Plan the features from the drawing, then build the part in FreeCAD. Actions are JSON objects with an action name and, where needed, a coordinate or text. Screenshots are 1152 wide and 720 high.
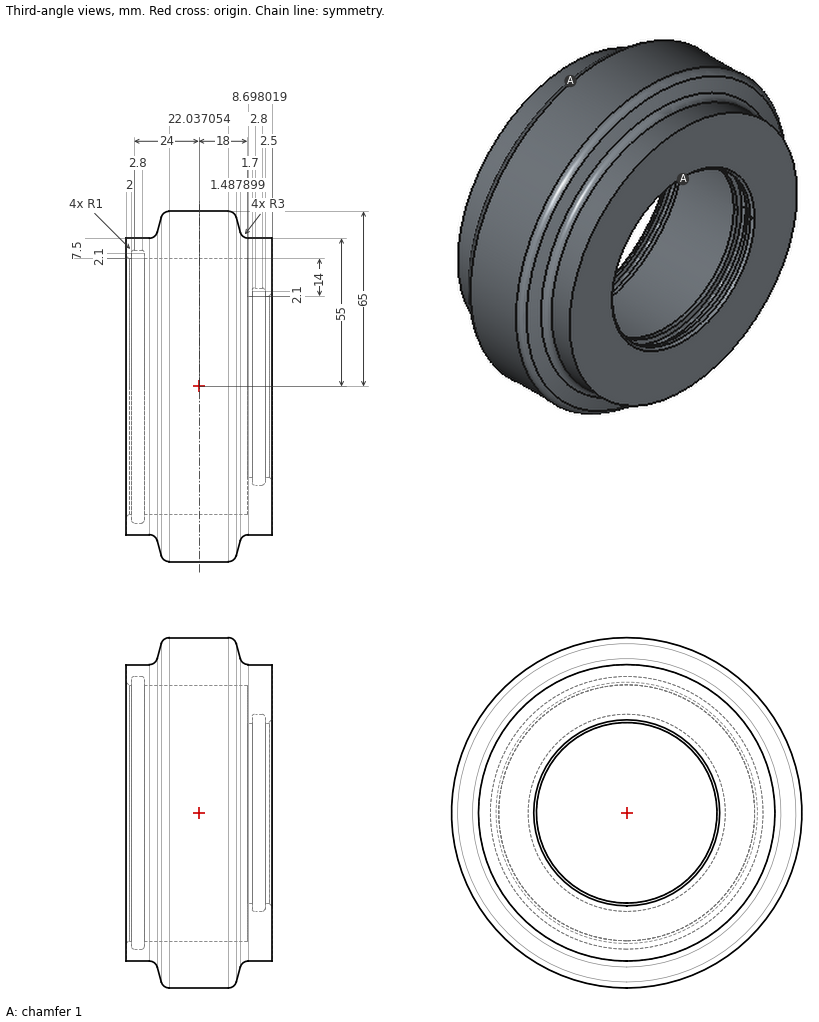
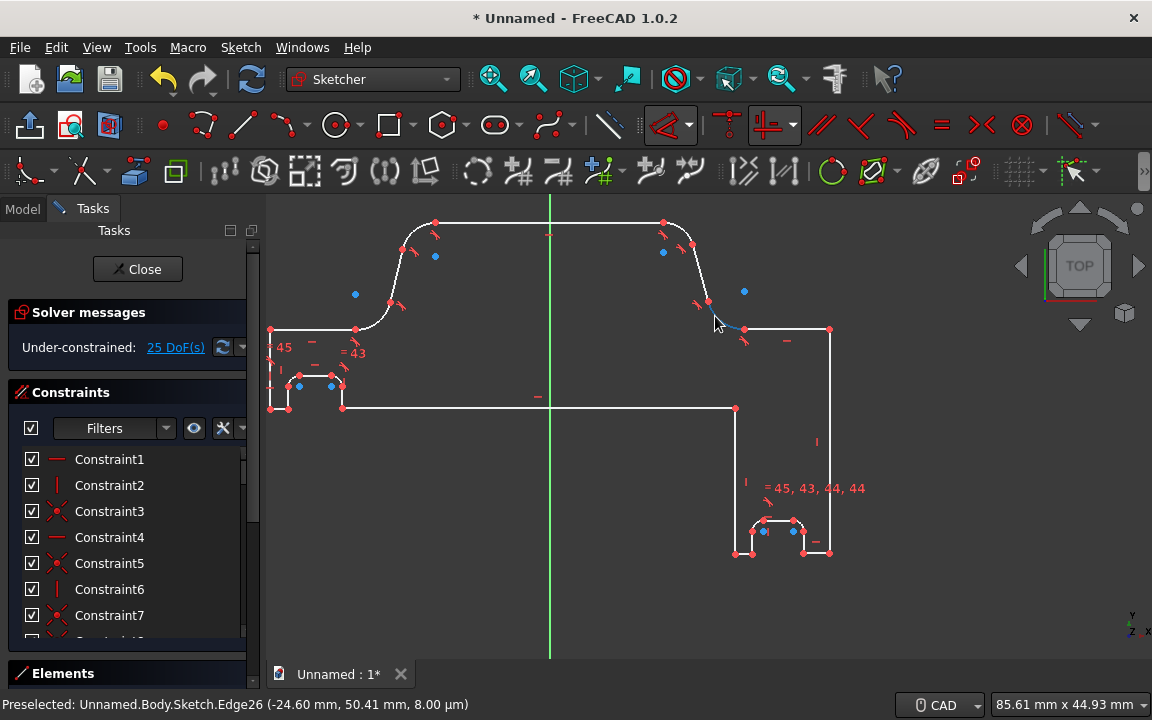
{"action": "left_click", "coordinate": [715, 315]}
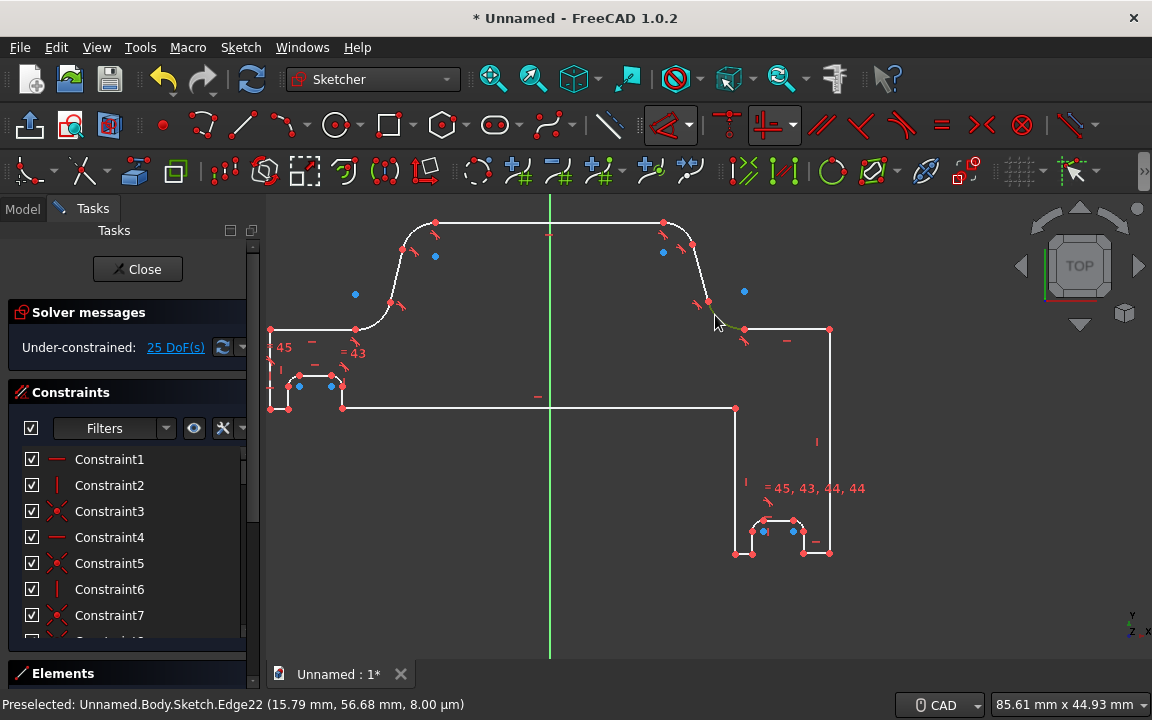
{"action": "left_click", "coordinate": [688, 235]}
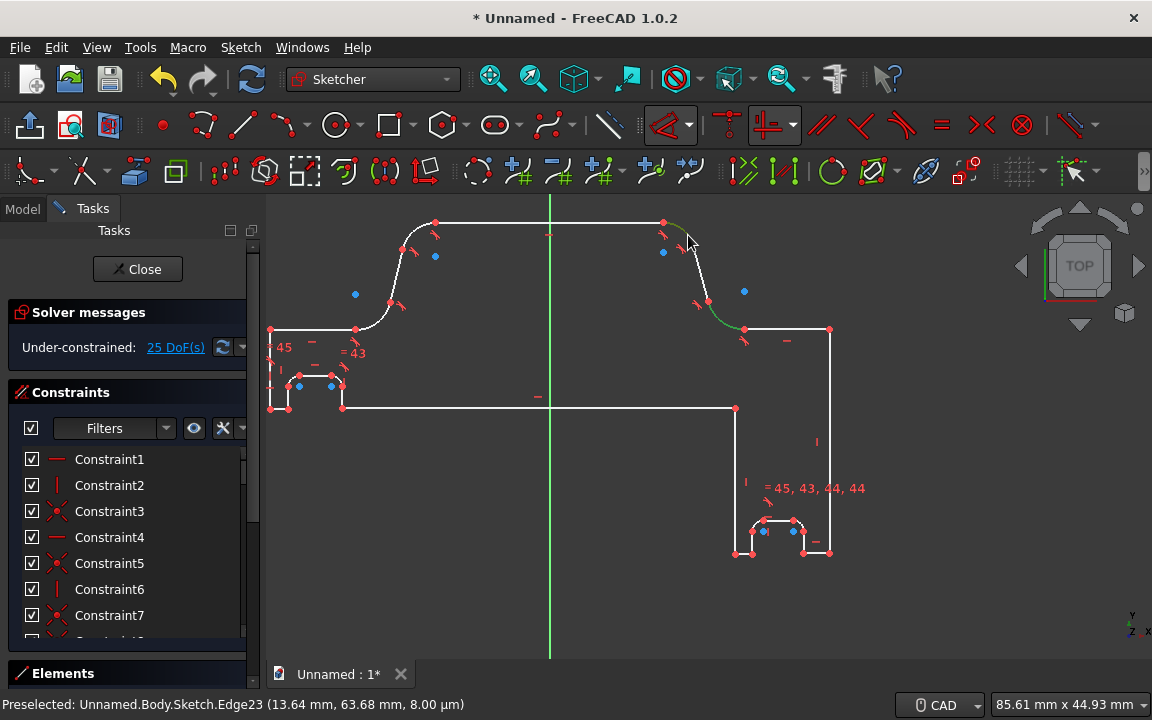
{"action": "left_click", "coordinate": [423, 226]}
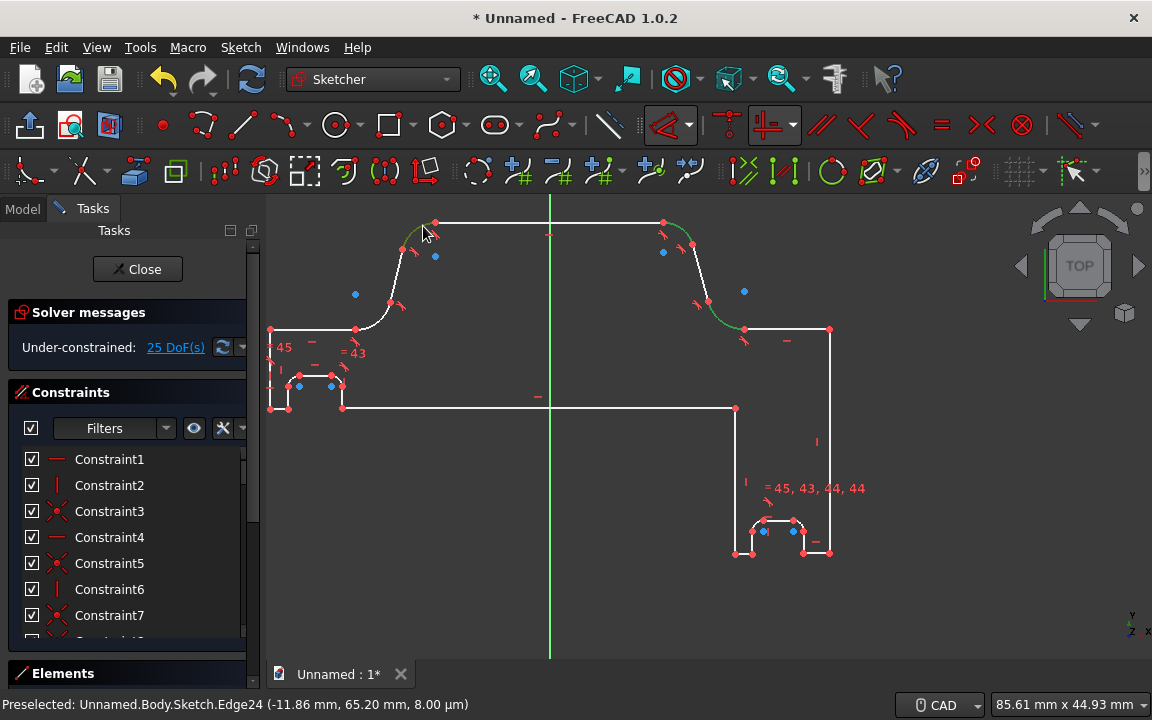
{"action": "left_click", "coordinate": [370, 327]}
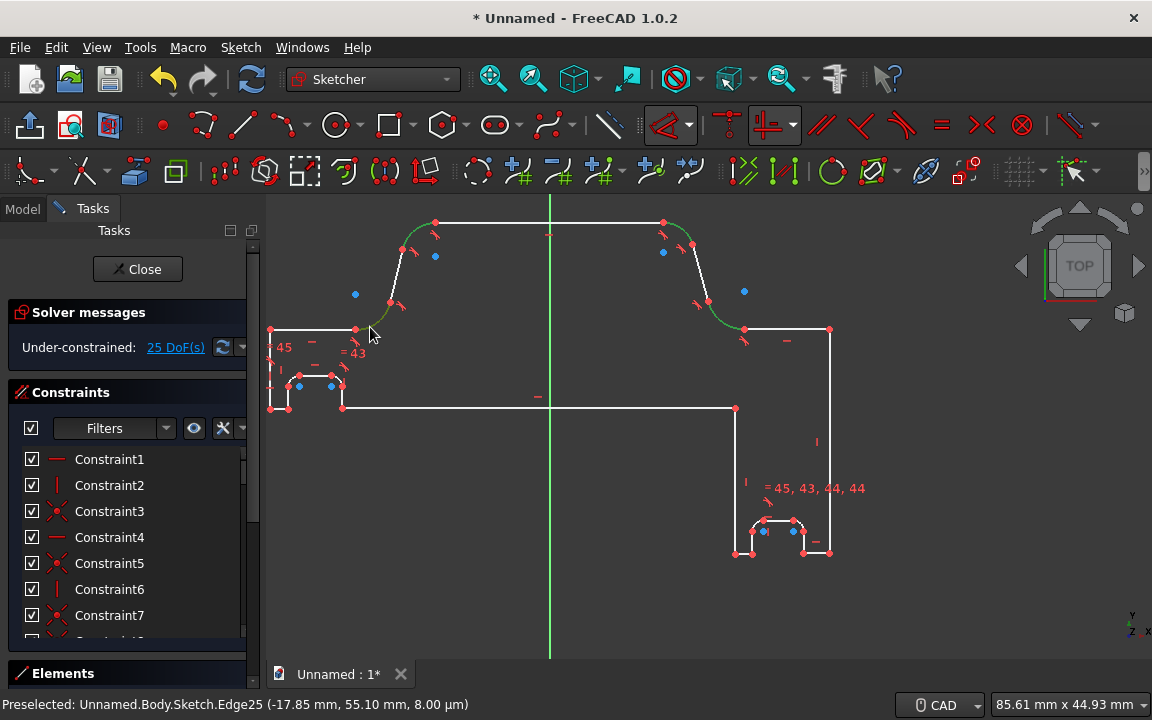
{"action": "left_click", "coordinate": [942, 126]}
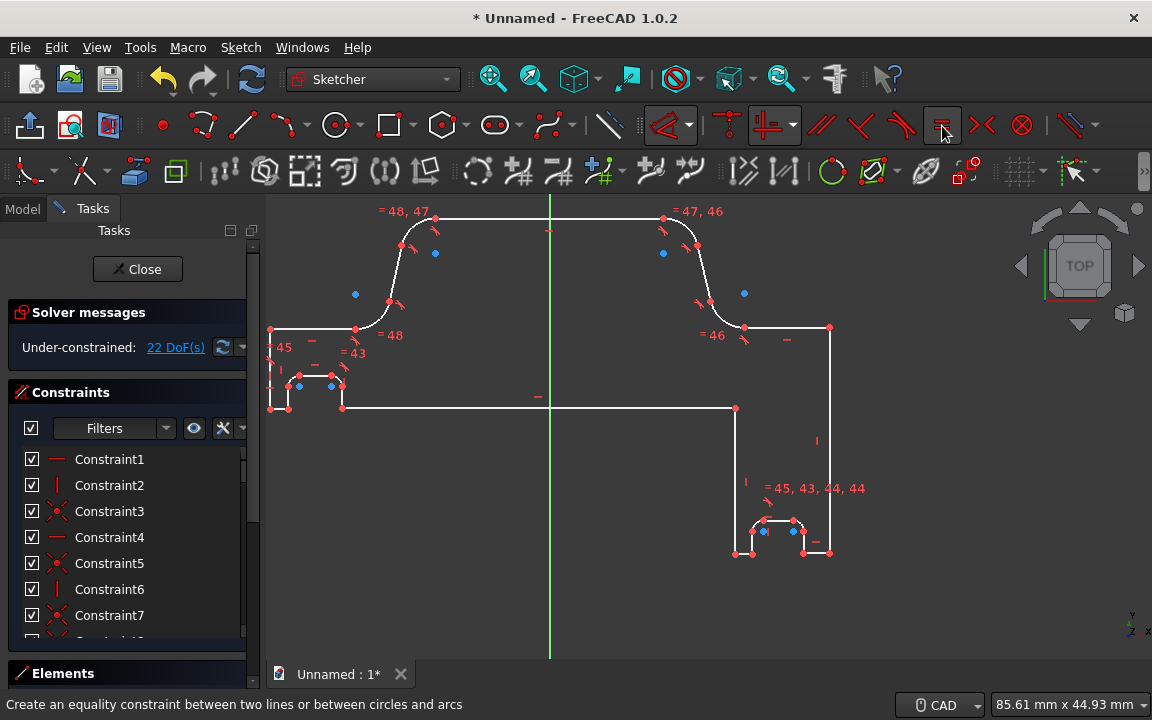
{"action": "left_click", "coordinate": [745, 293]}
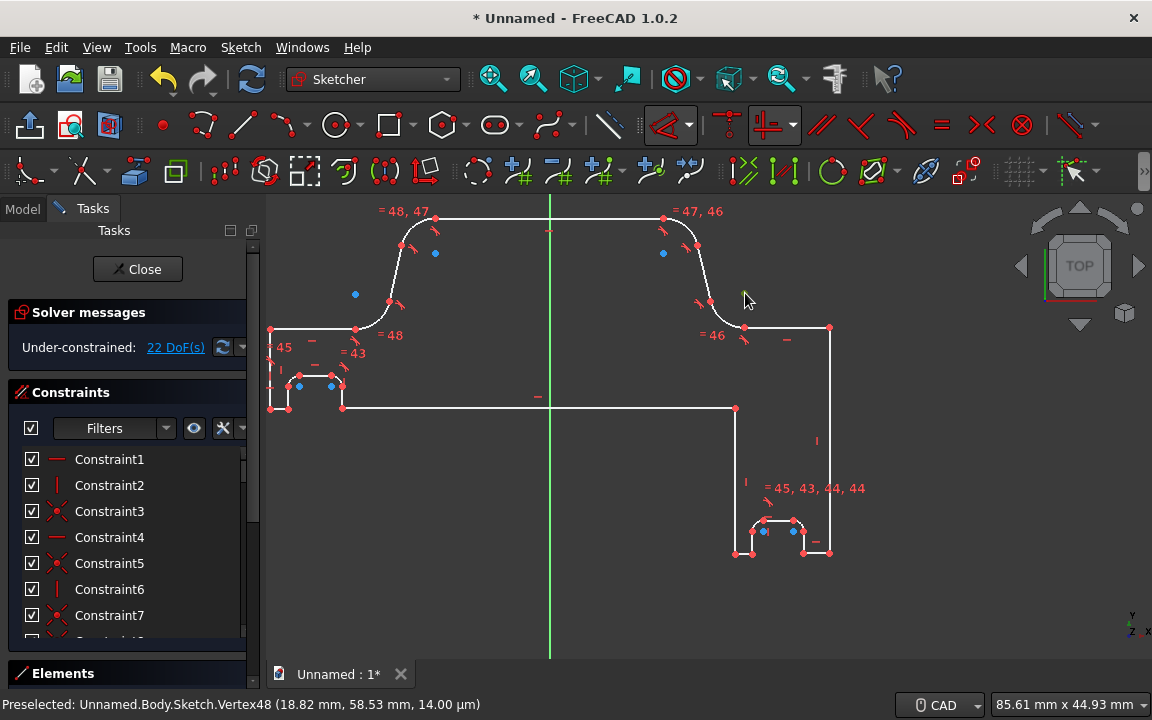
{"action": "left_click", "coordinate": [356, 294]}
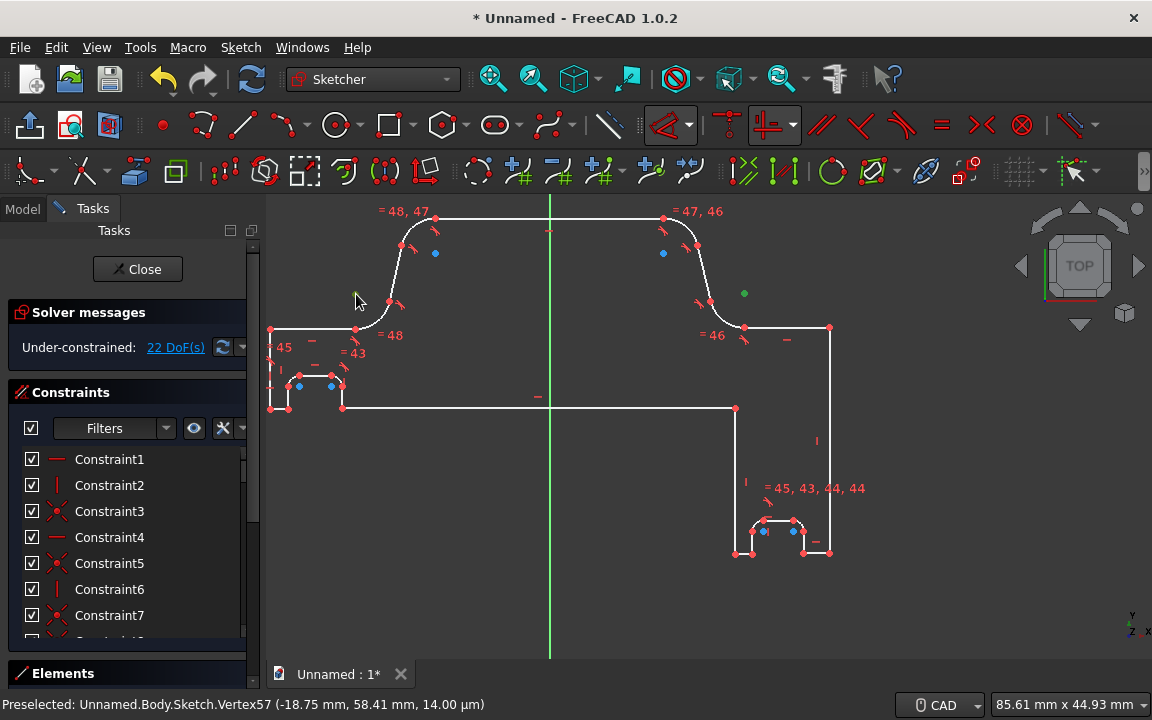
{"action": "left_click", "coordinate": [550, 602]}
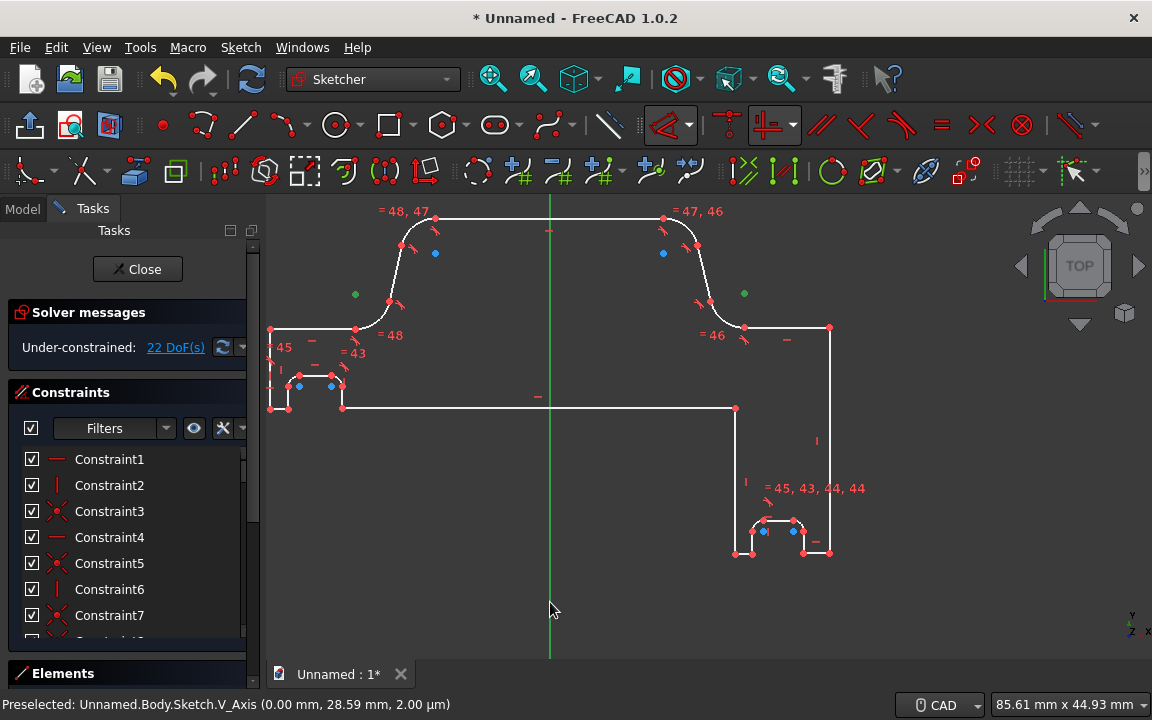
{"action": "key", "text": "s"}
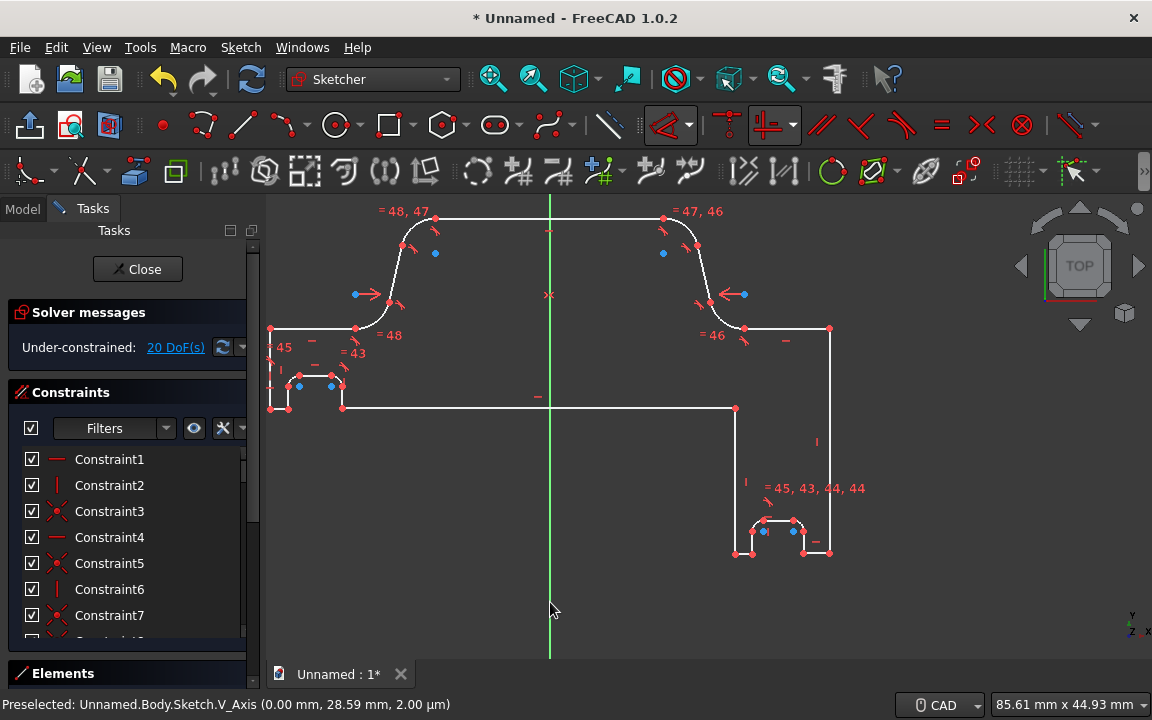
{"action": "scroll", "coordinate": [339, 379], "scroll_direction": "up", "scroll_amount": 7}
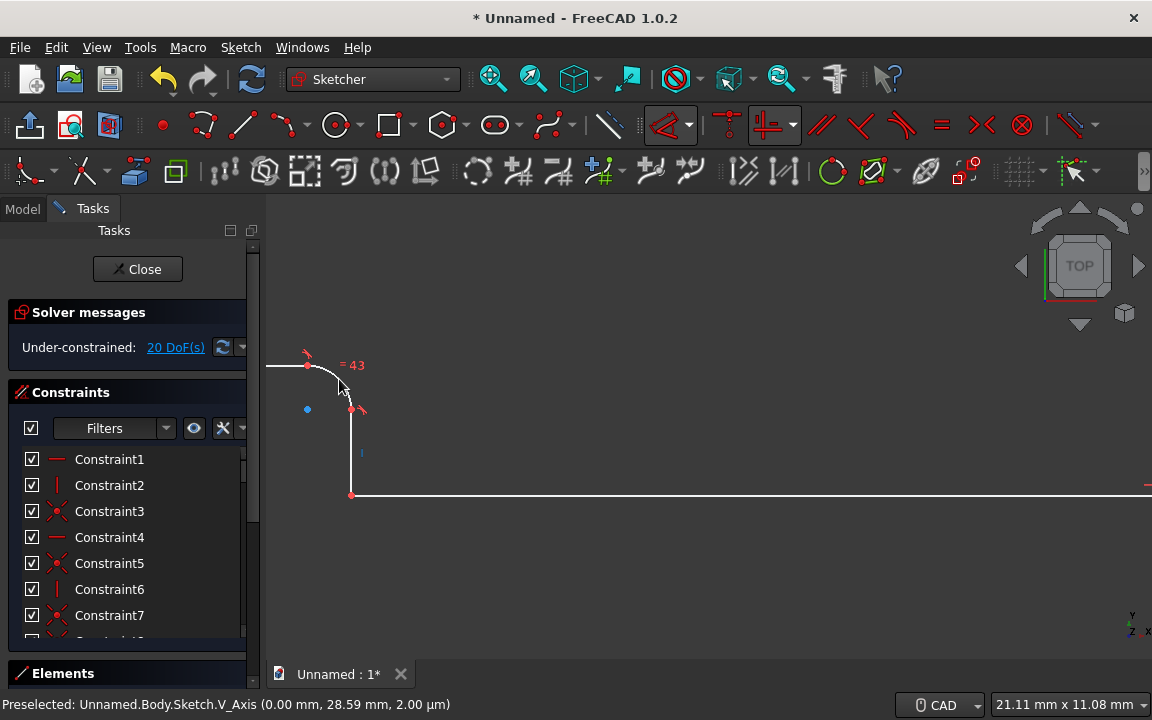
{"action": "left_click", "coordinate": [338, 378]}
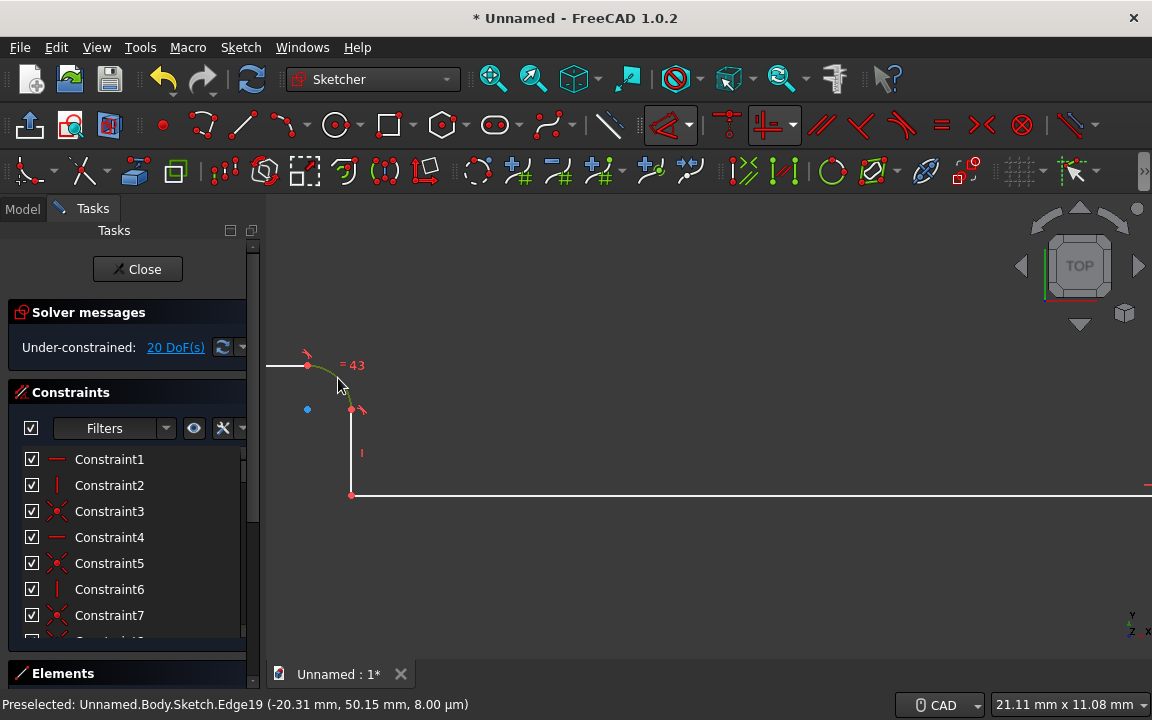
{"action": "key", "text": "k r"}